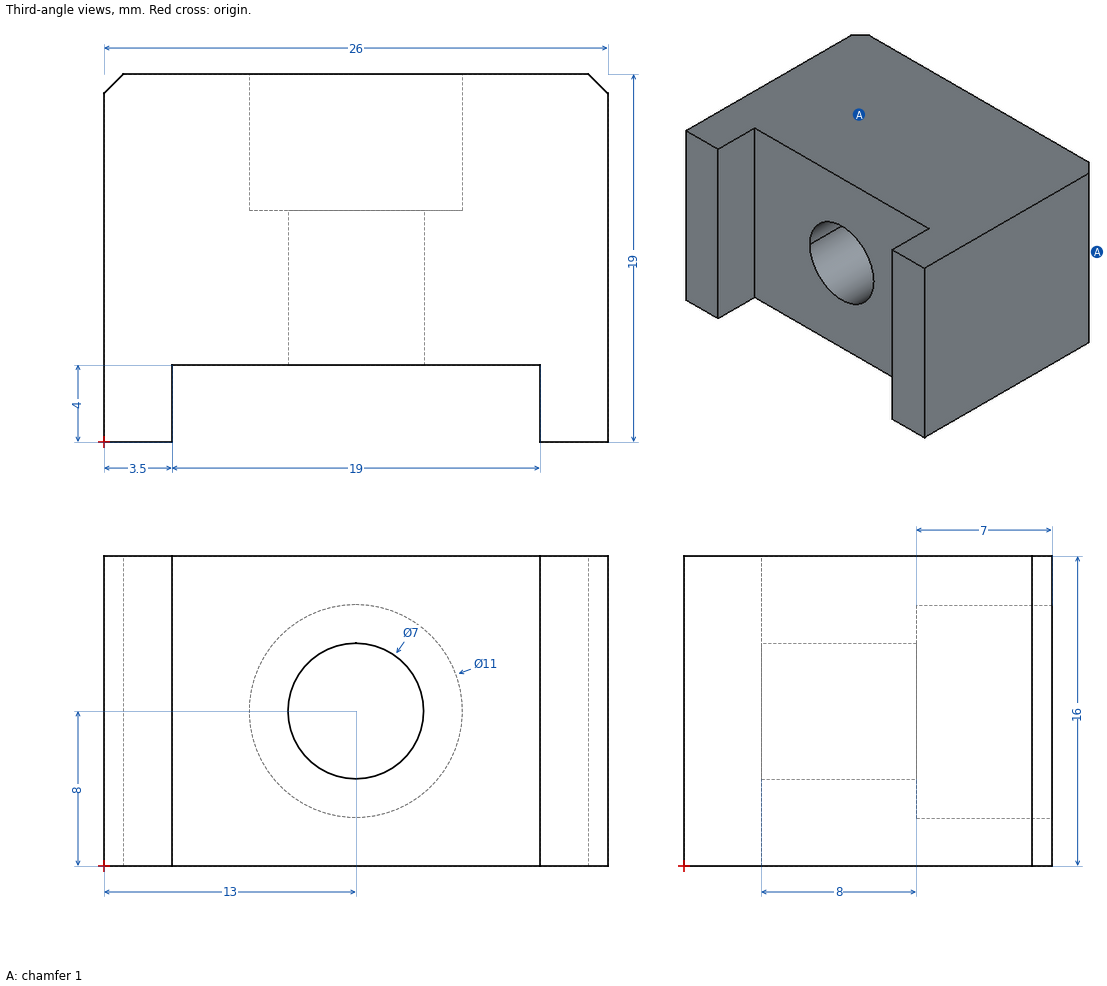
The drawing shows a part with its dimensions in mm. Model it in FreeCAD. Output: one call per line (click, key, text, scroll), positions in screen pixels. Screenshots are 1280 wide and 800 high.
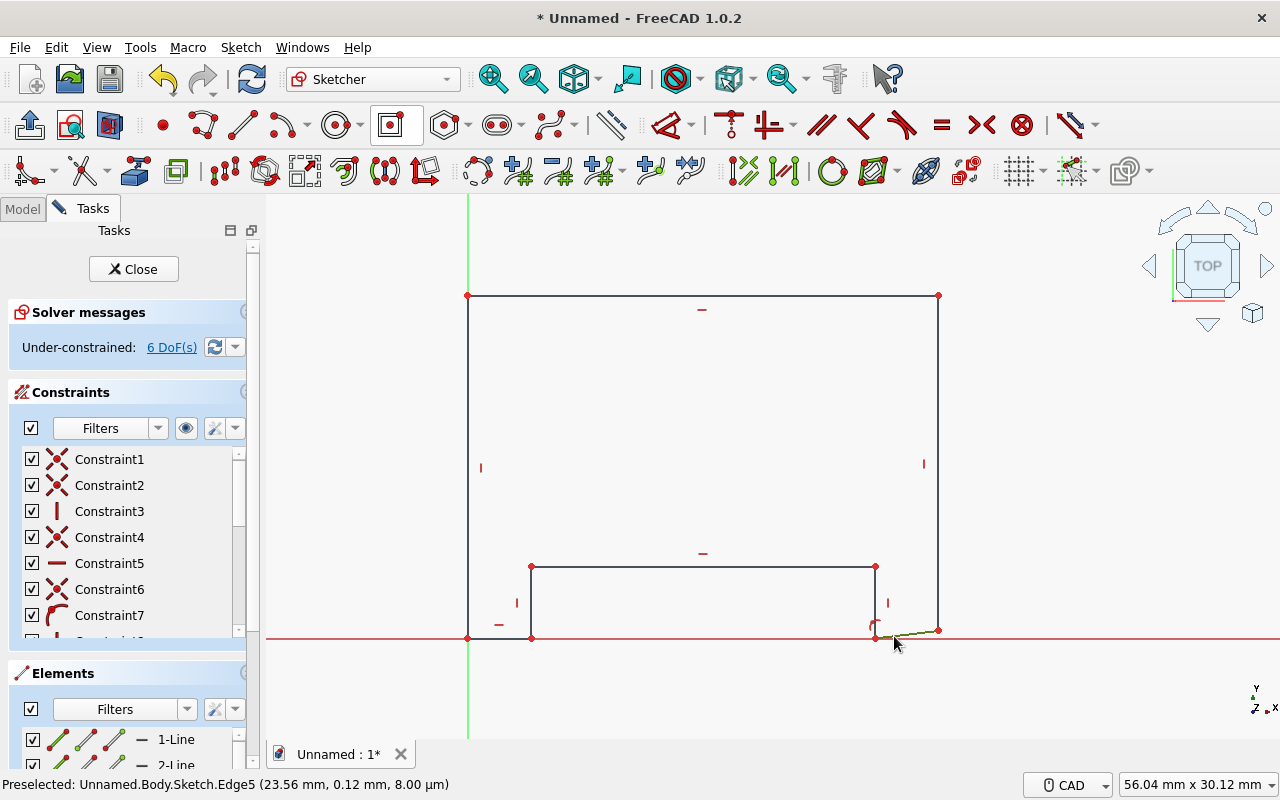
key(h)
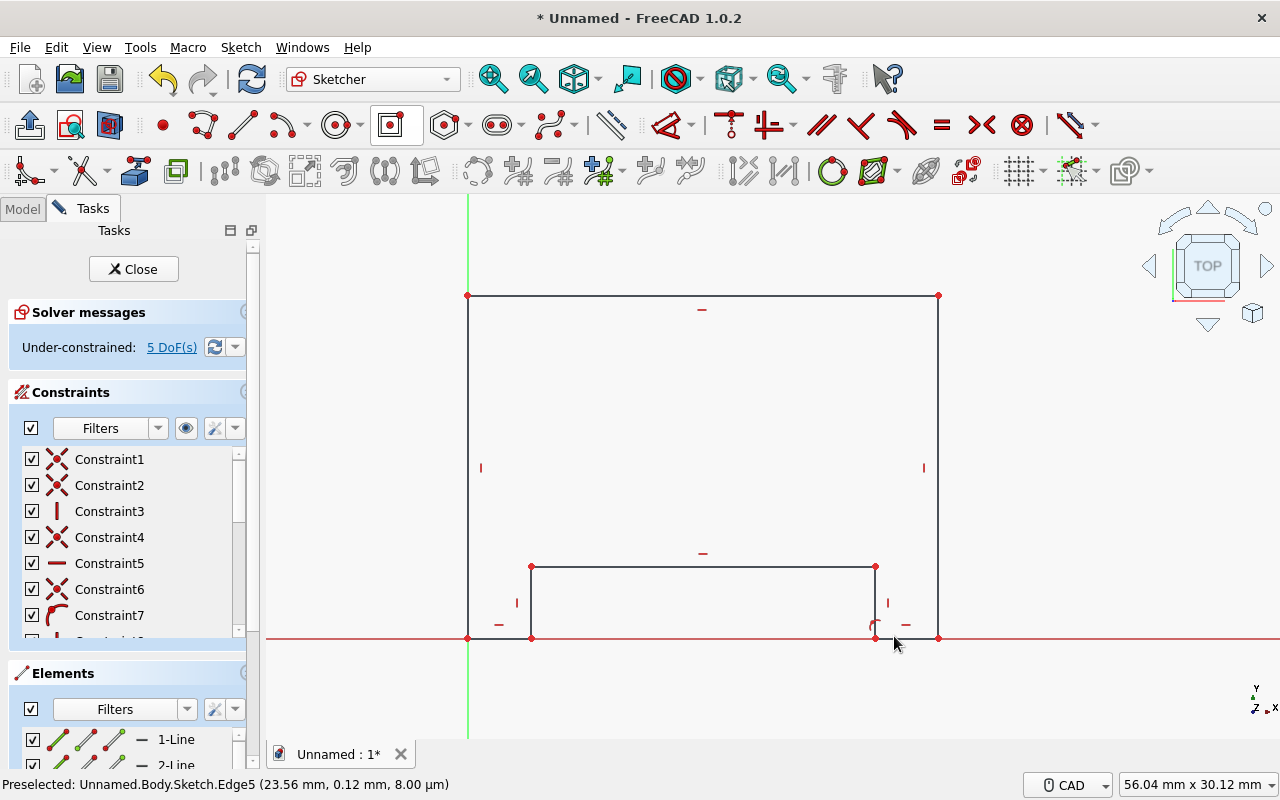
click(531, 617)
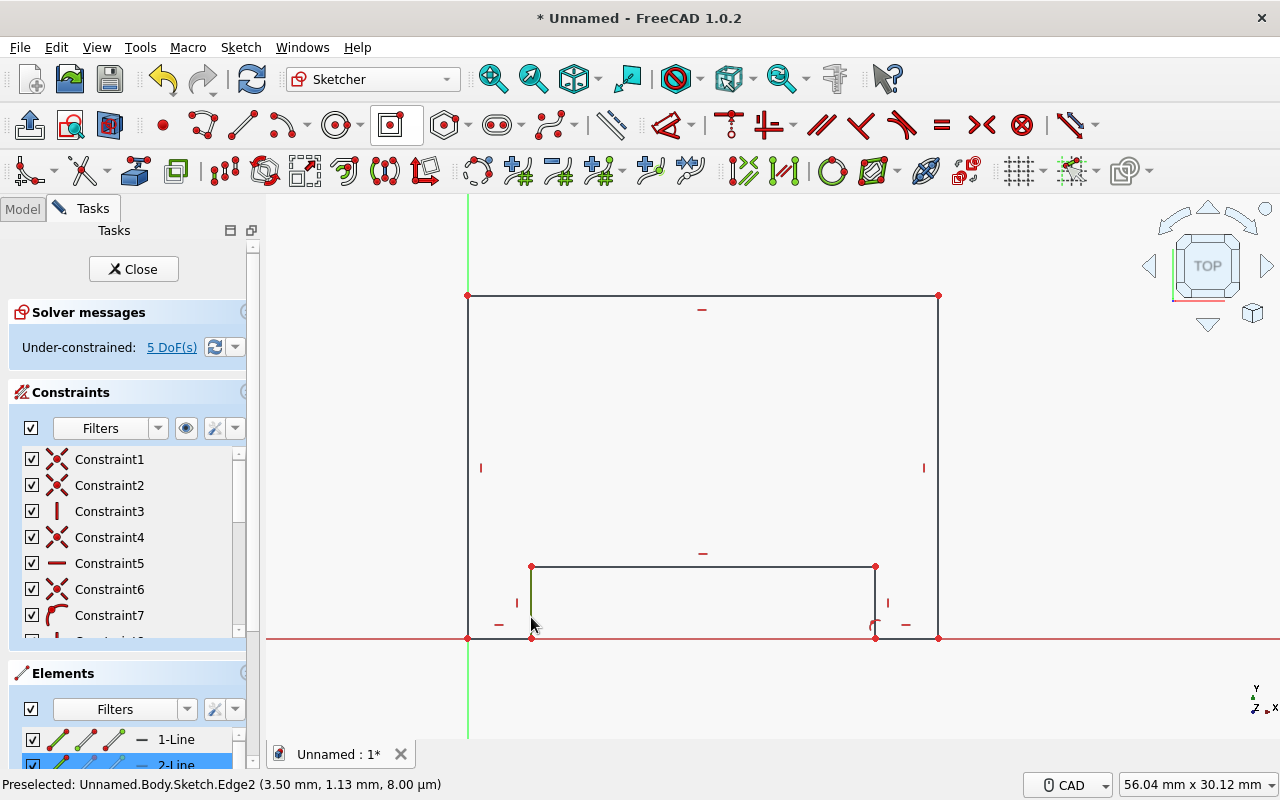
click(694, 126)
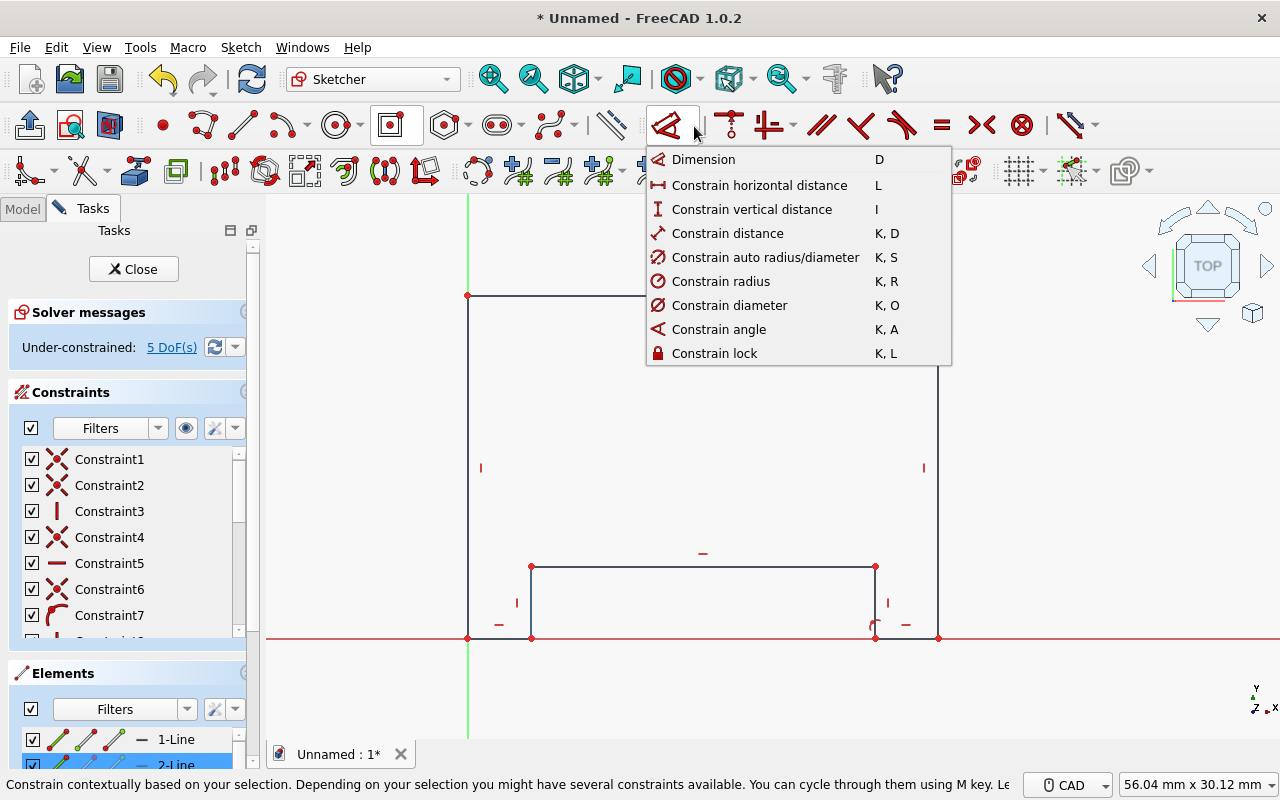
click(799, 209)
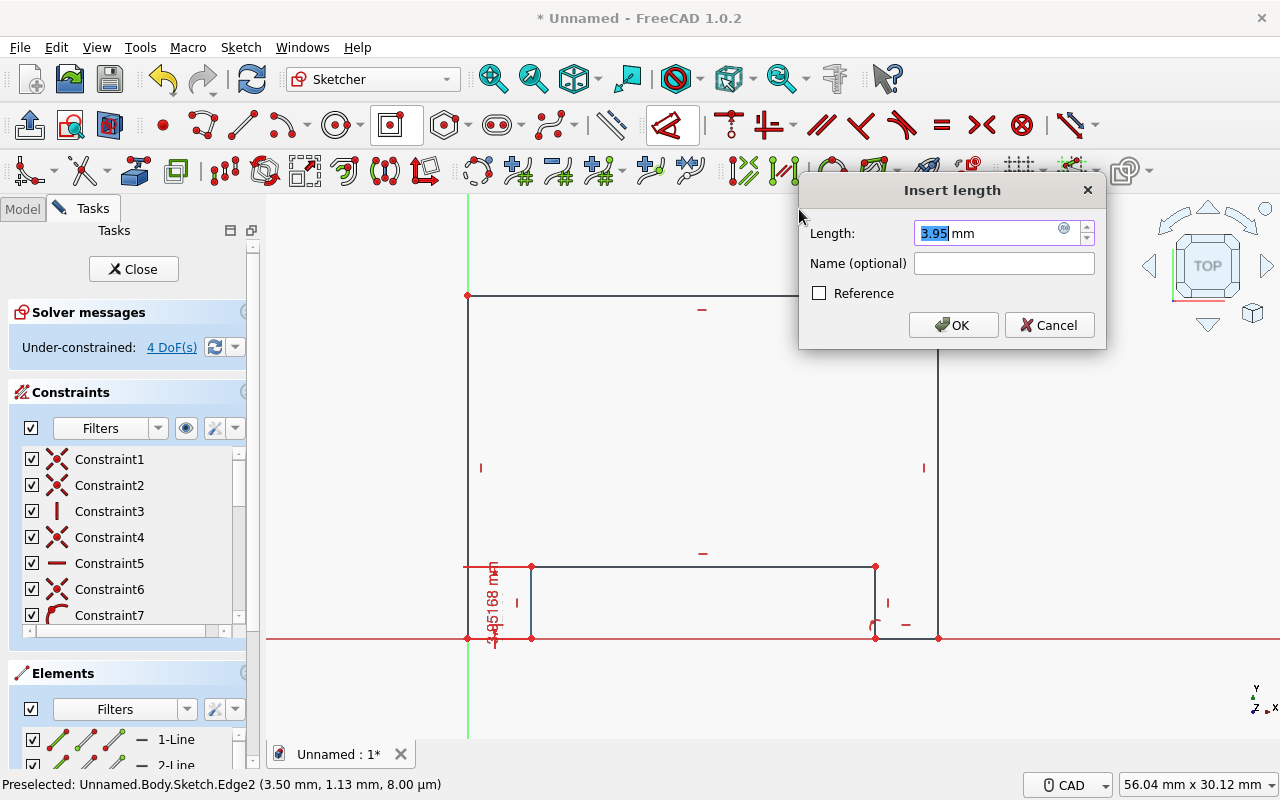
text(4)
key(Return)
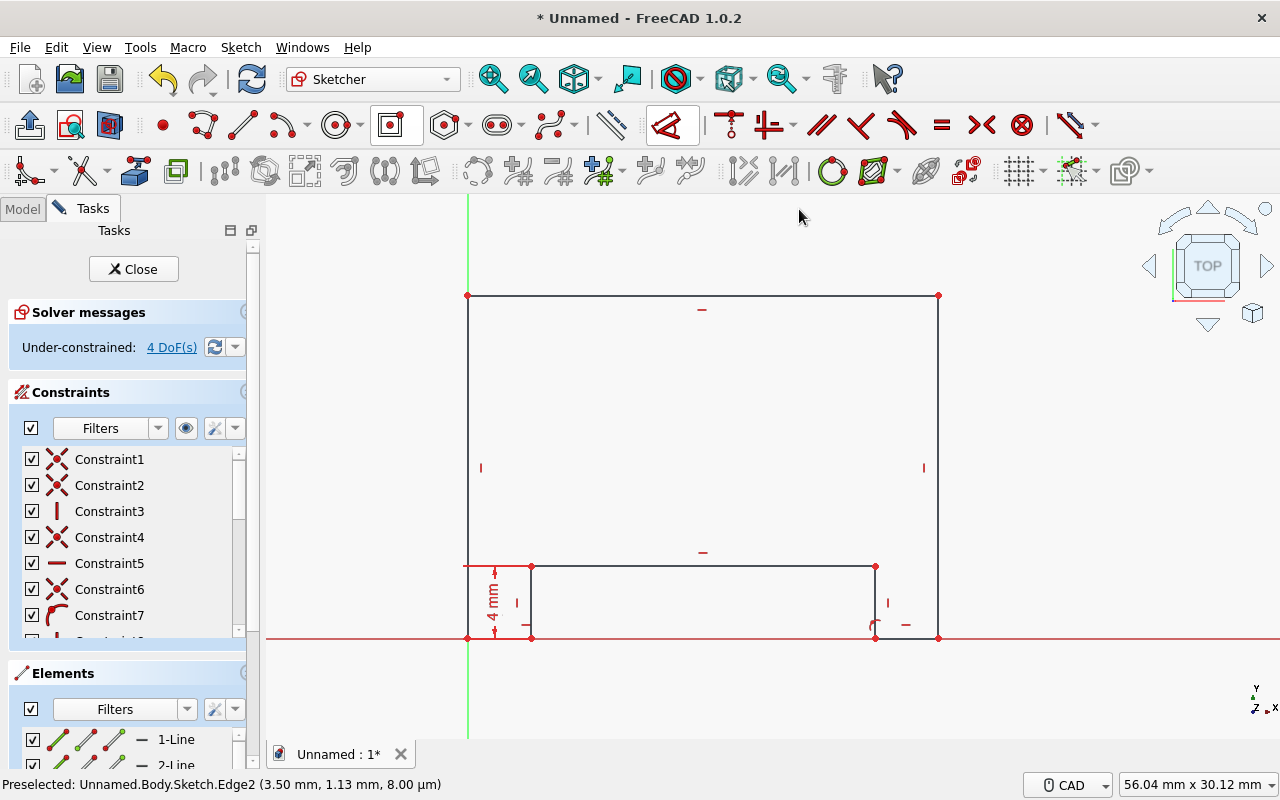
click(634, 566)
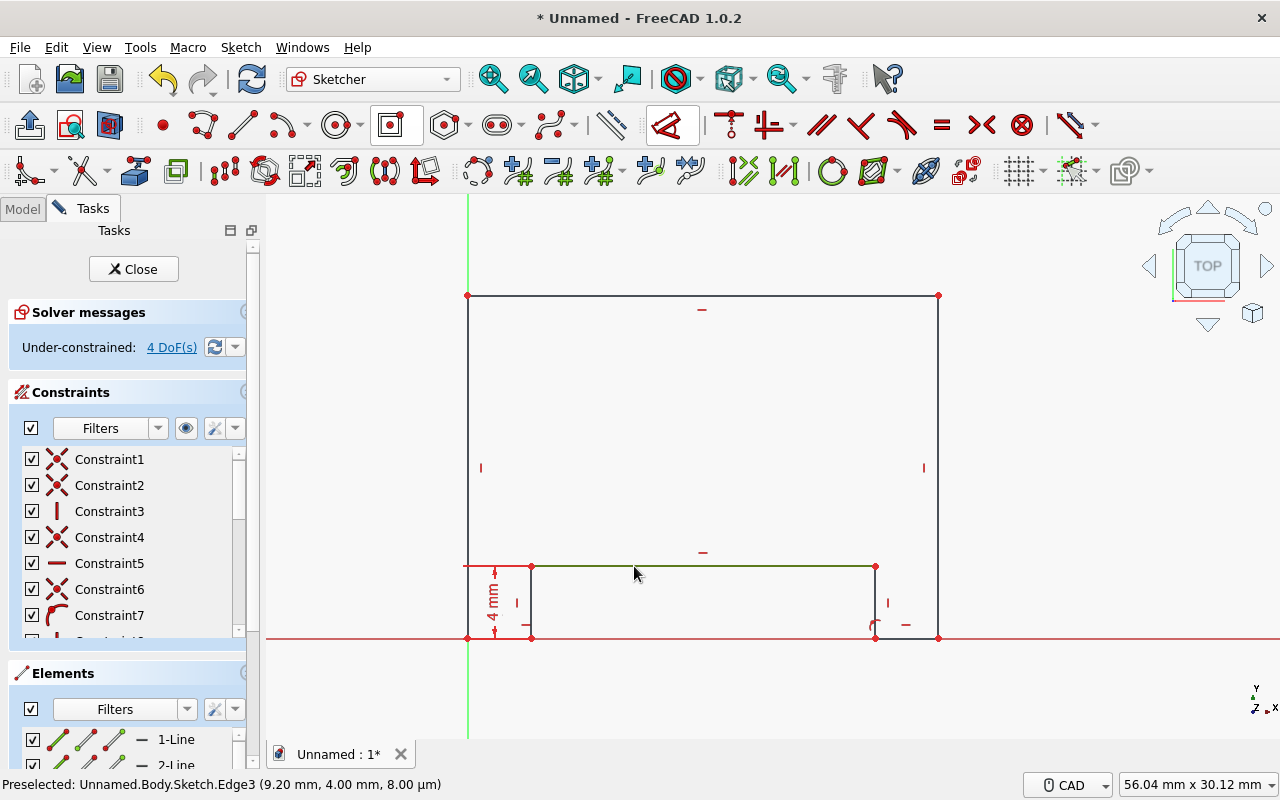
key(l)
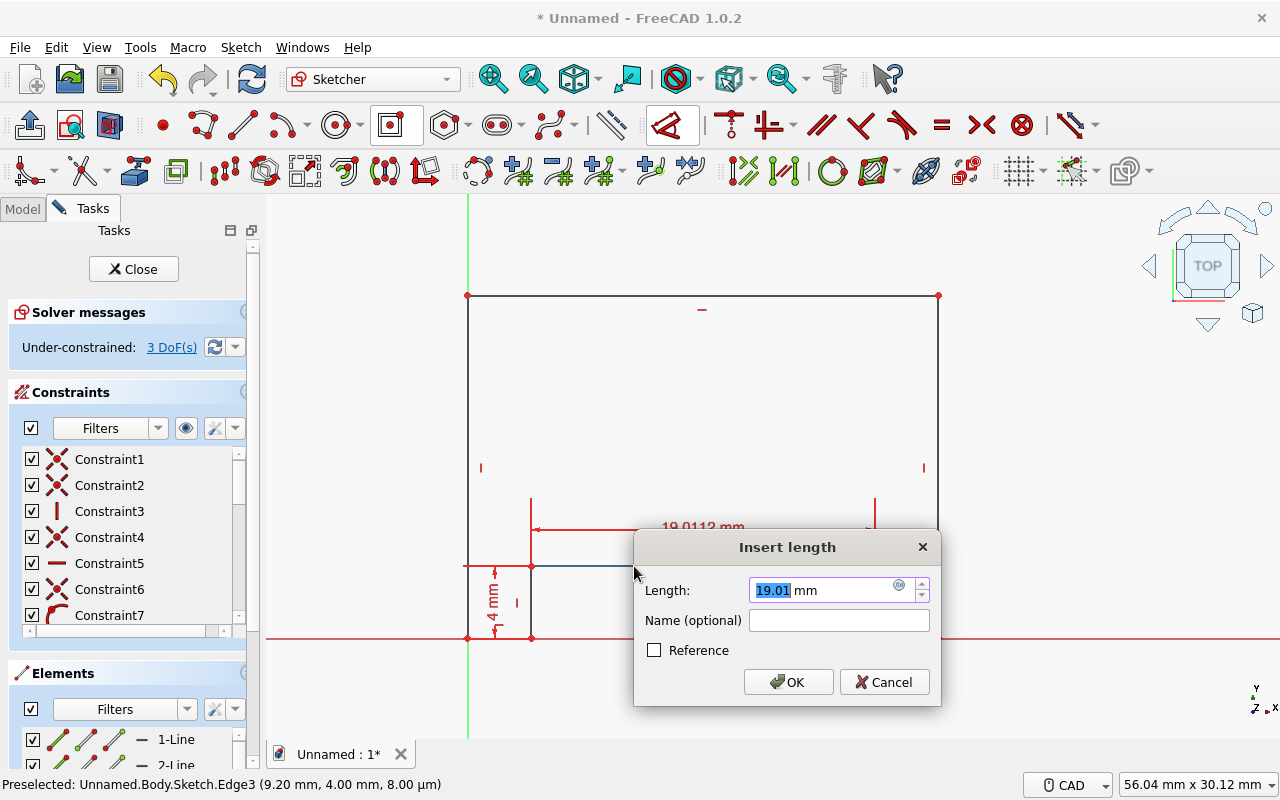
text(19)
key(Return)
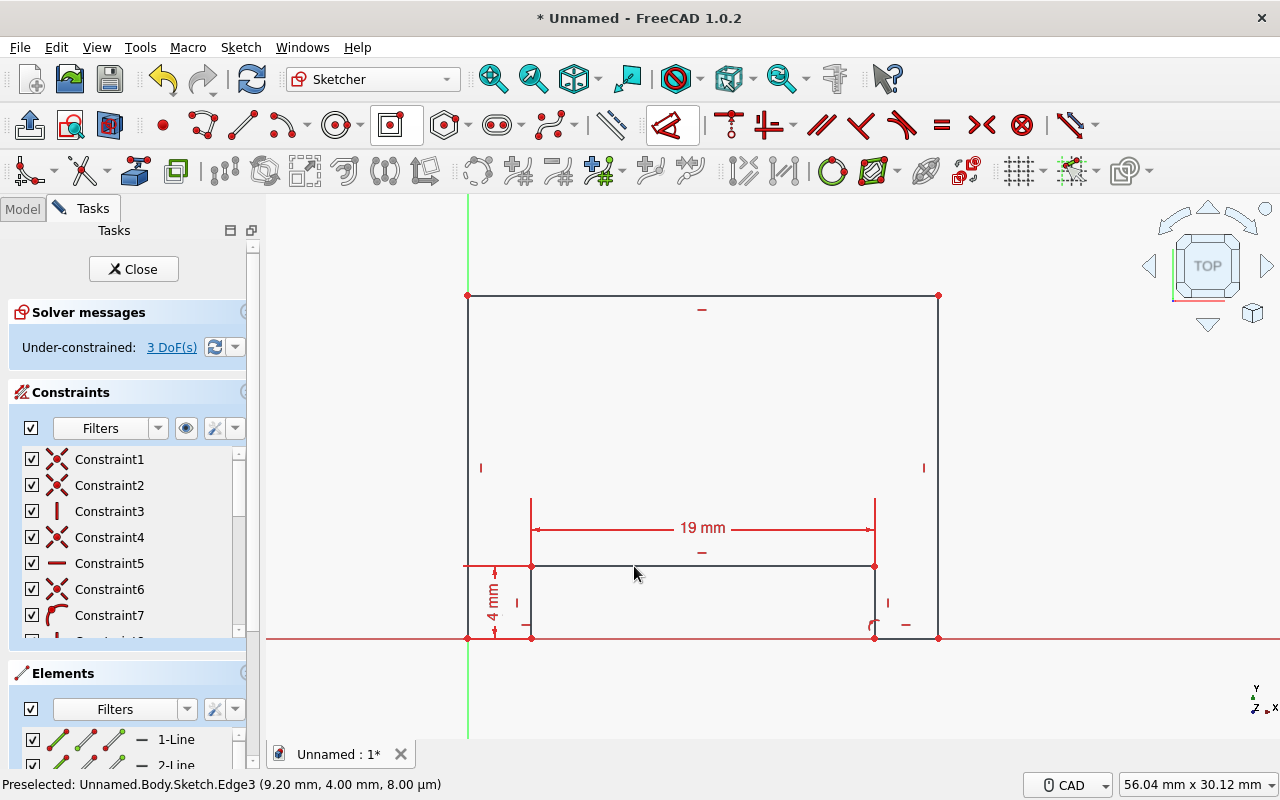
click(938, 536)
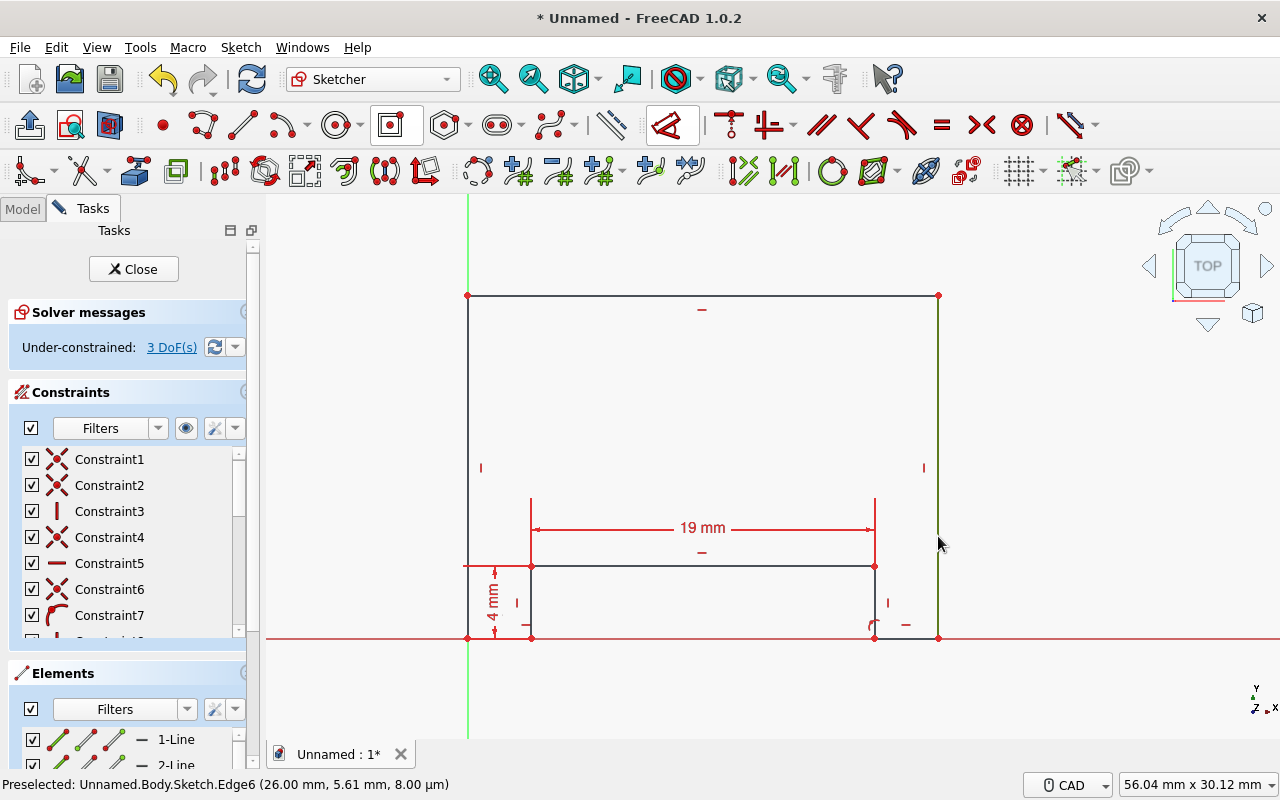
key(i)